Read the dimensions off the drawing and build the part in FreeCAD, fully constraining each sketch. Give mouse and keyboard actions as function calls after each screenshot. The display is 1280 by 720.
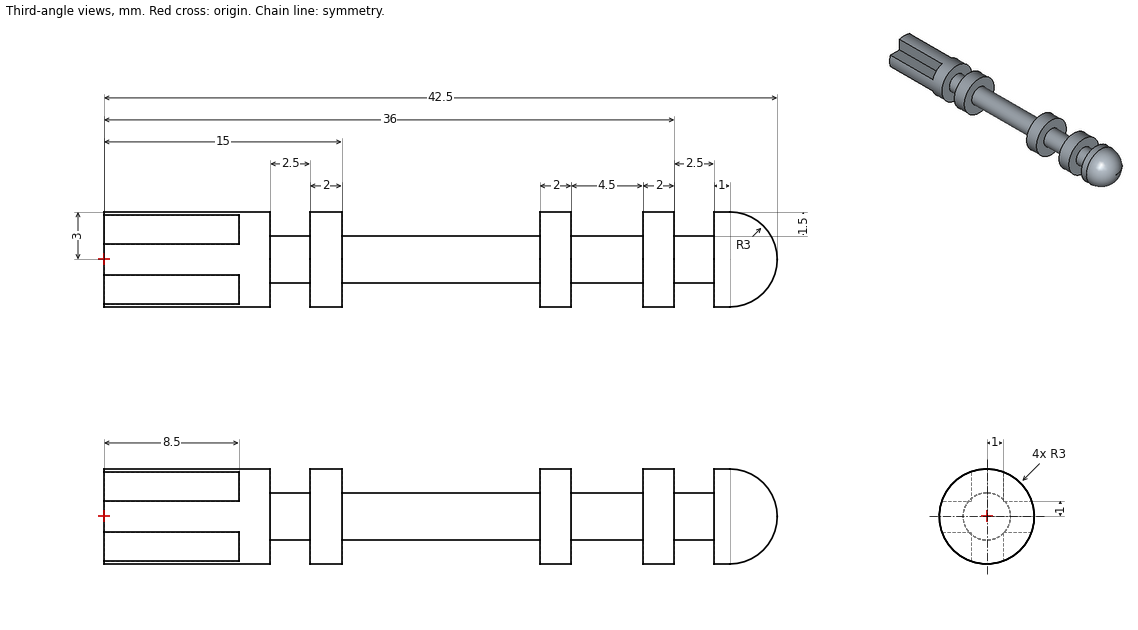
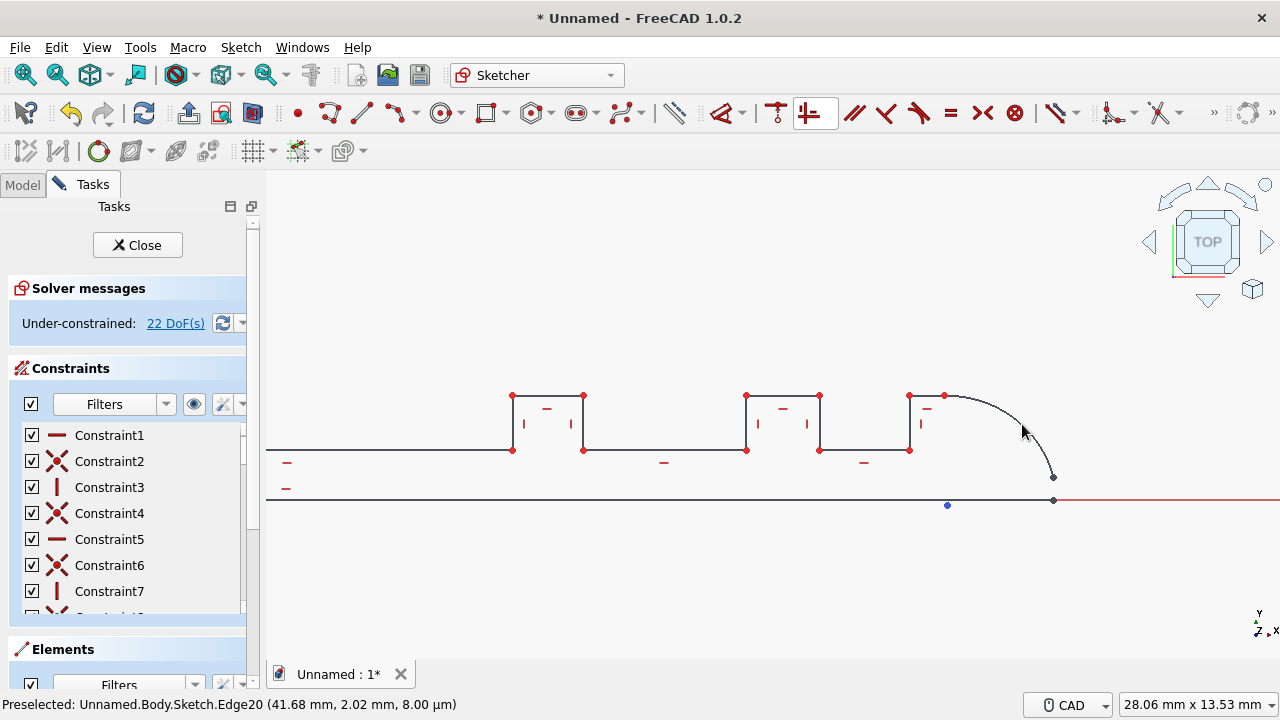
scroll(934, 396, up, 2)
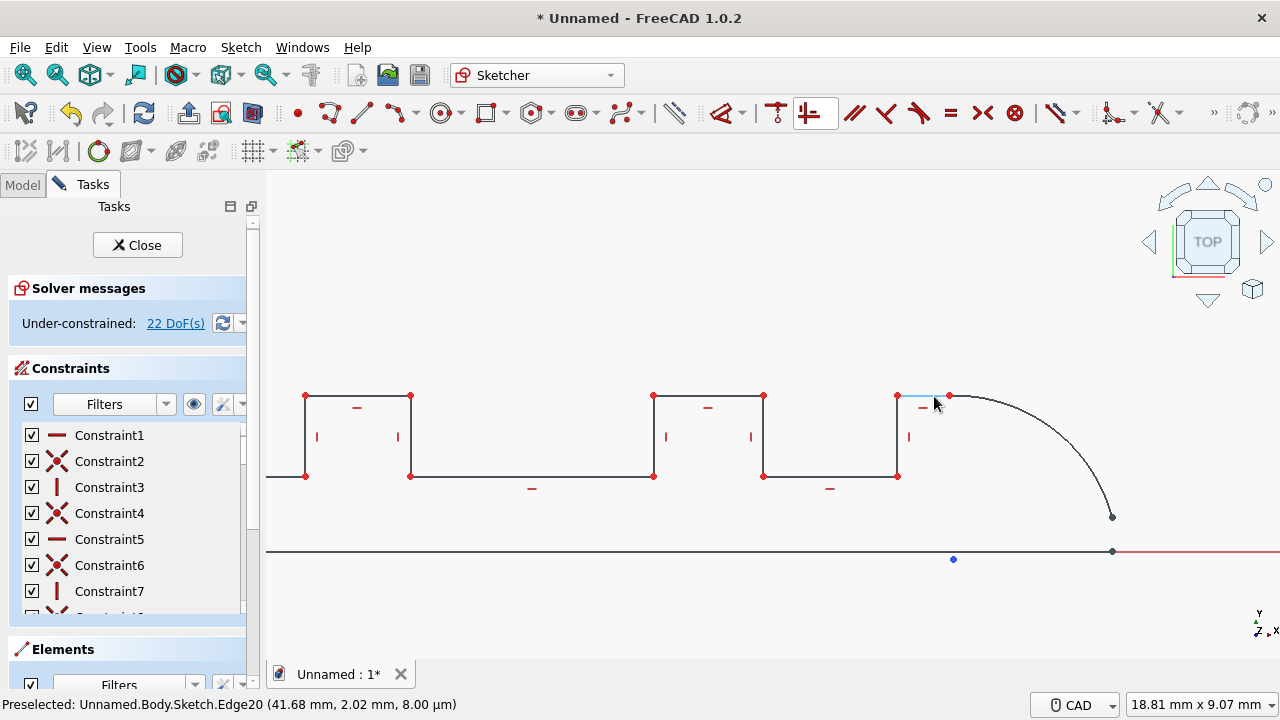
click(934, 396)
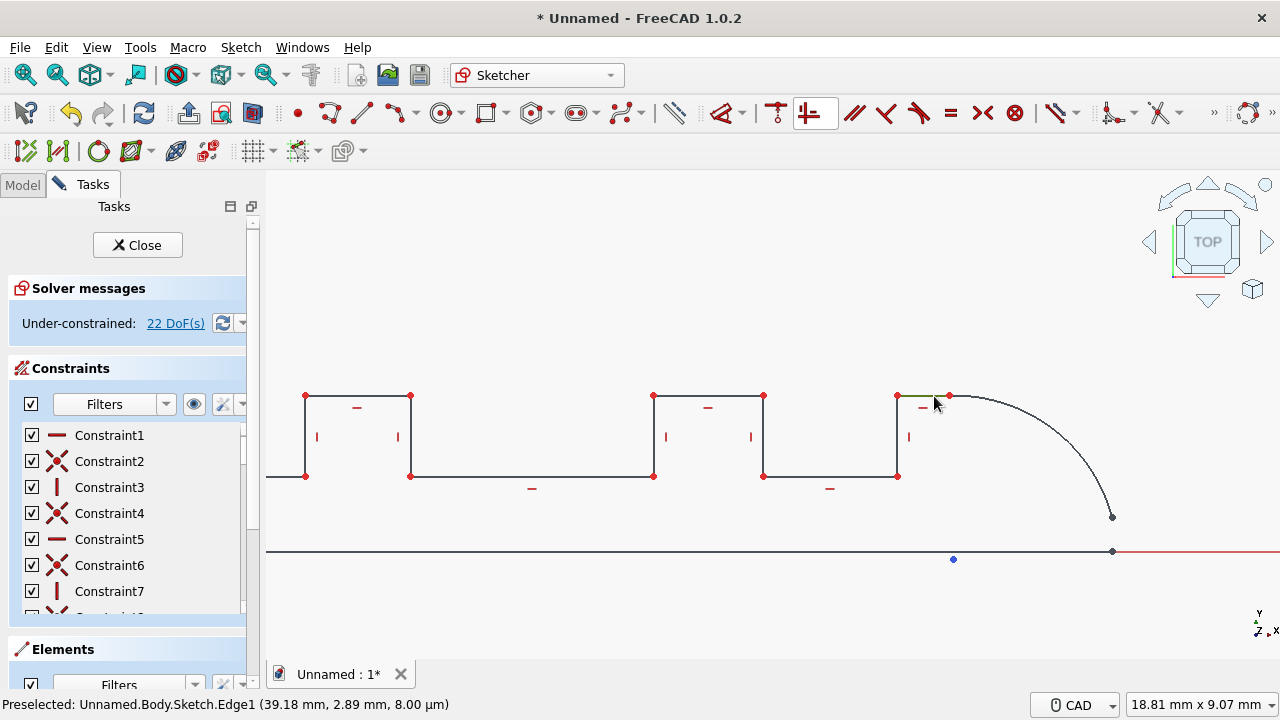
scroll(946, 396, down, 7)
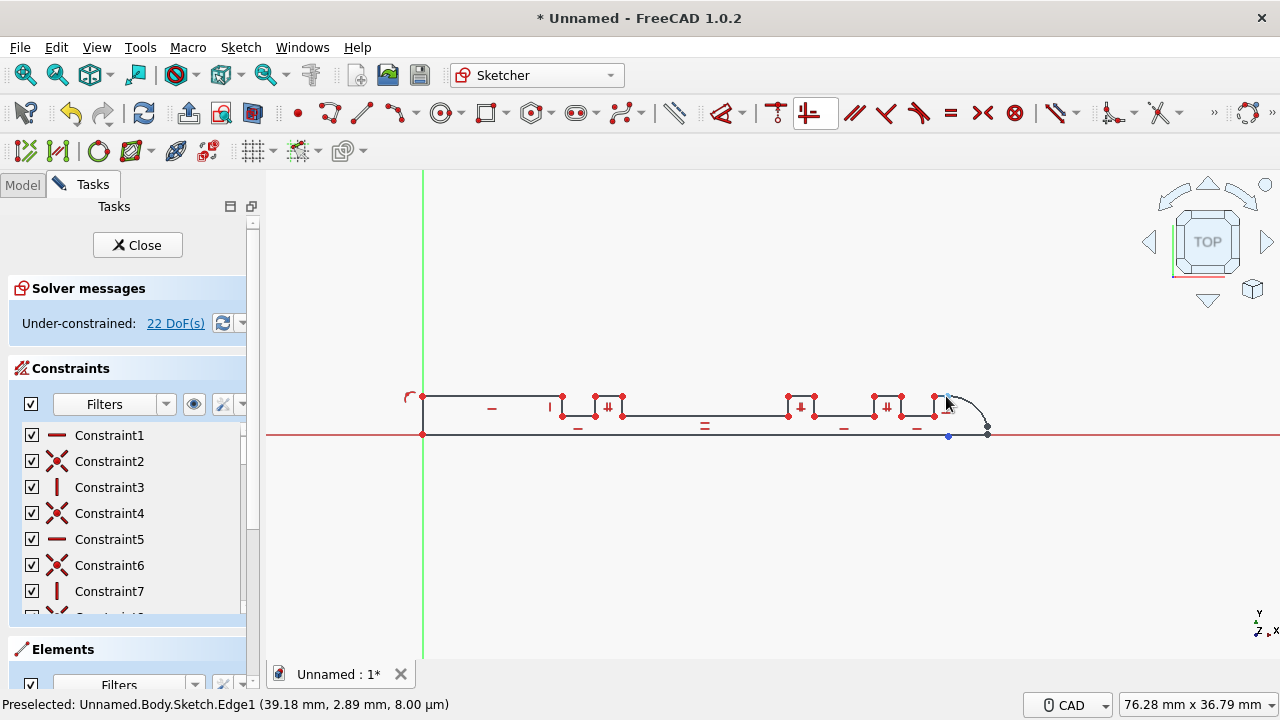
click(980, 412)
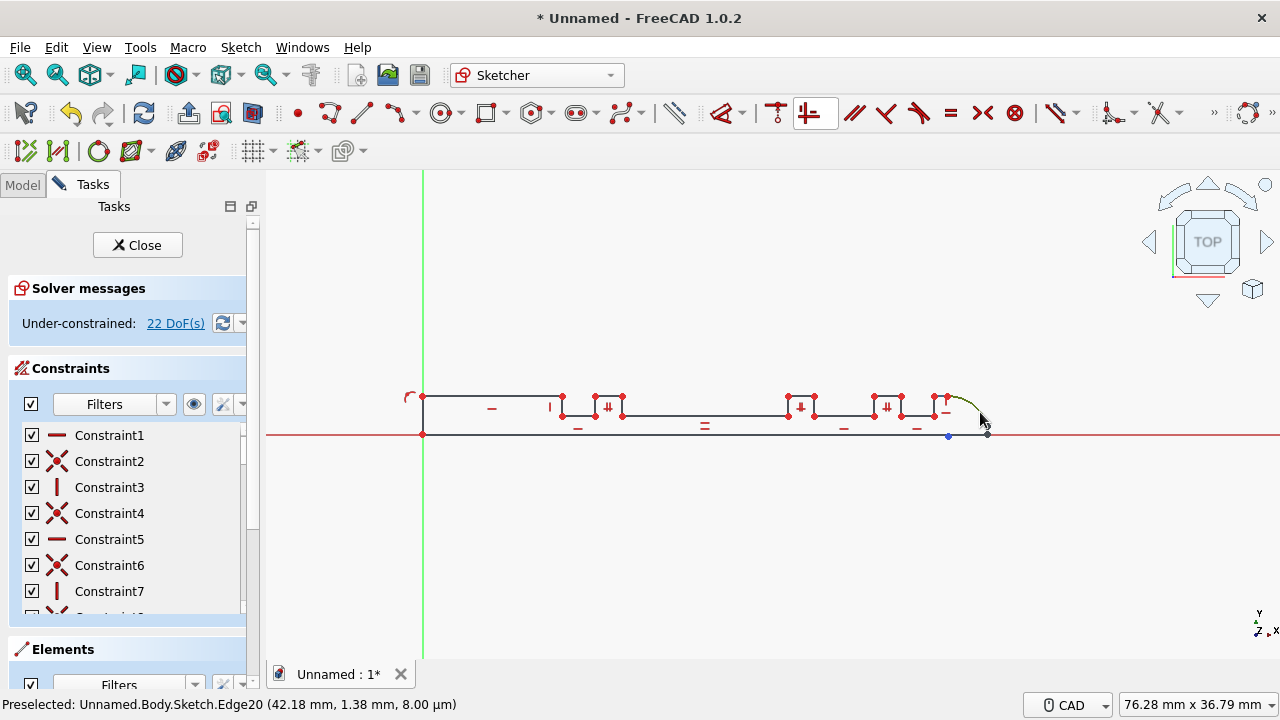
click(920, 114)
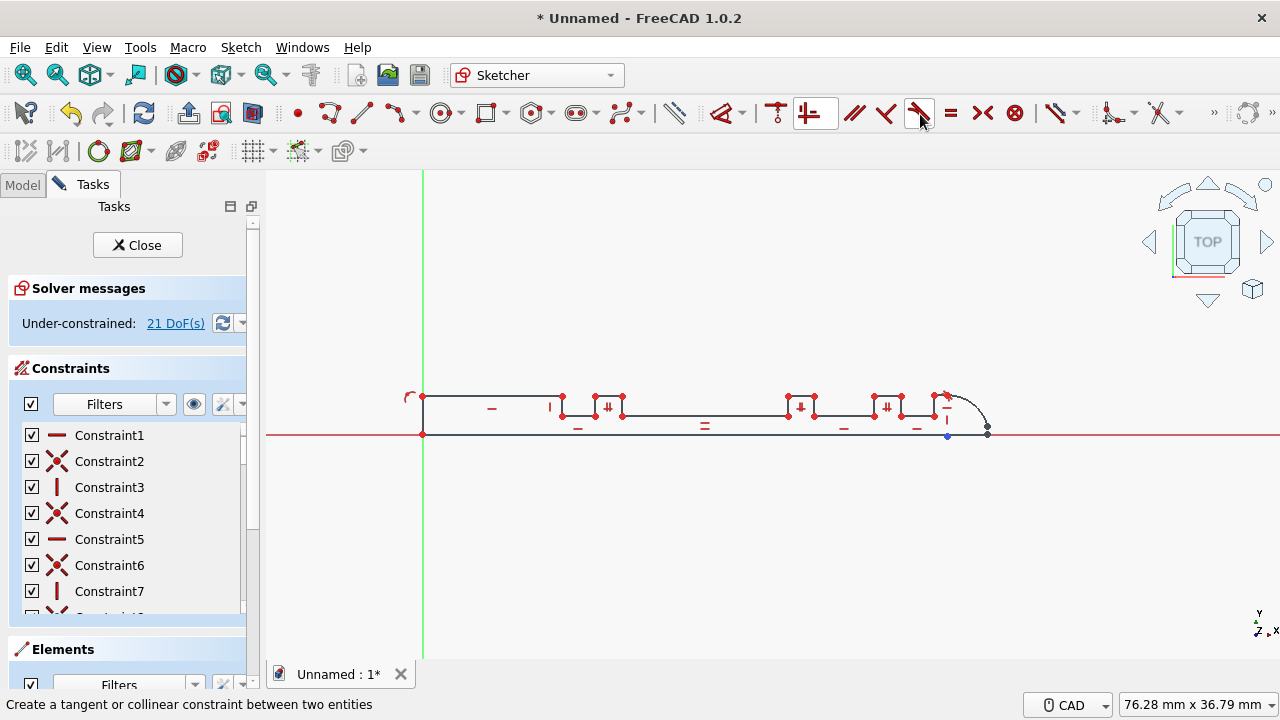
click(947, 437)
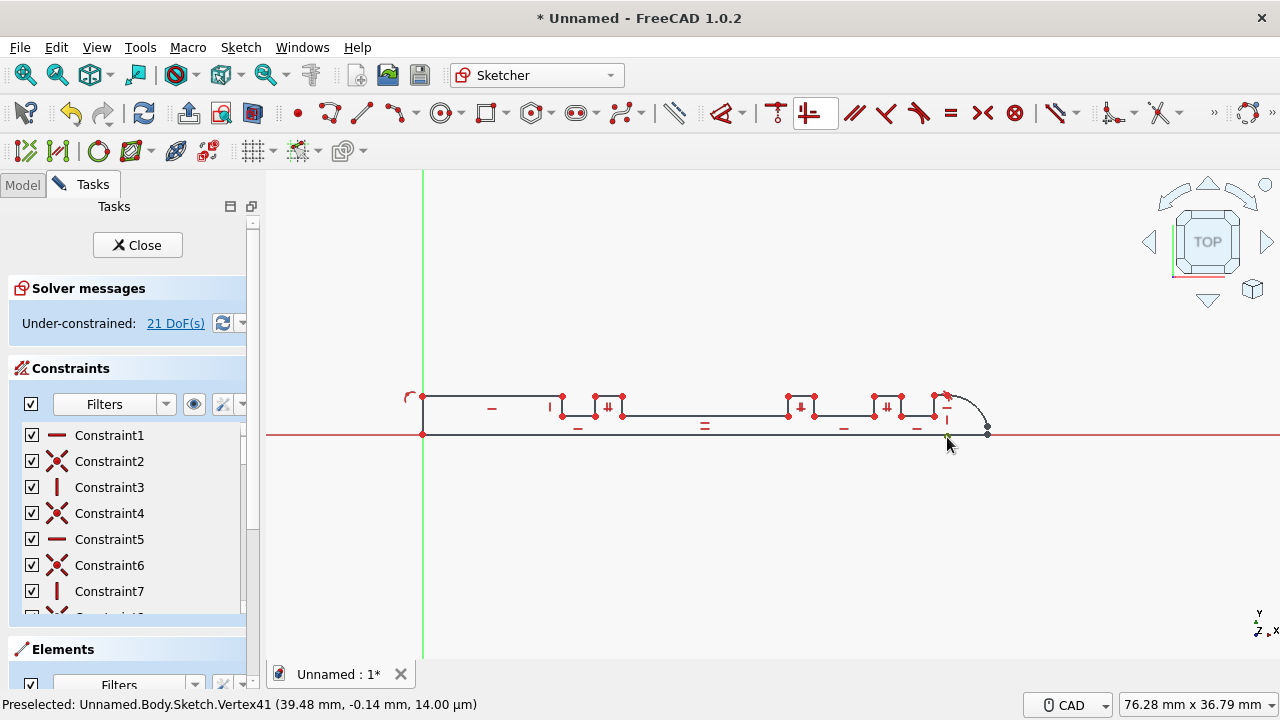
click(353, 435)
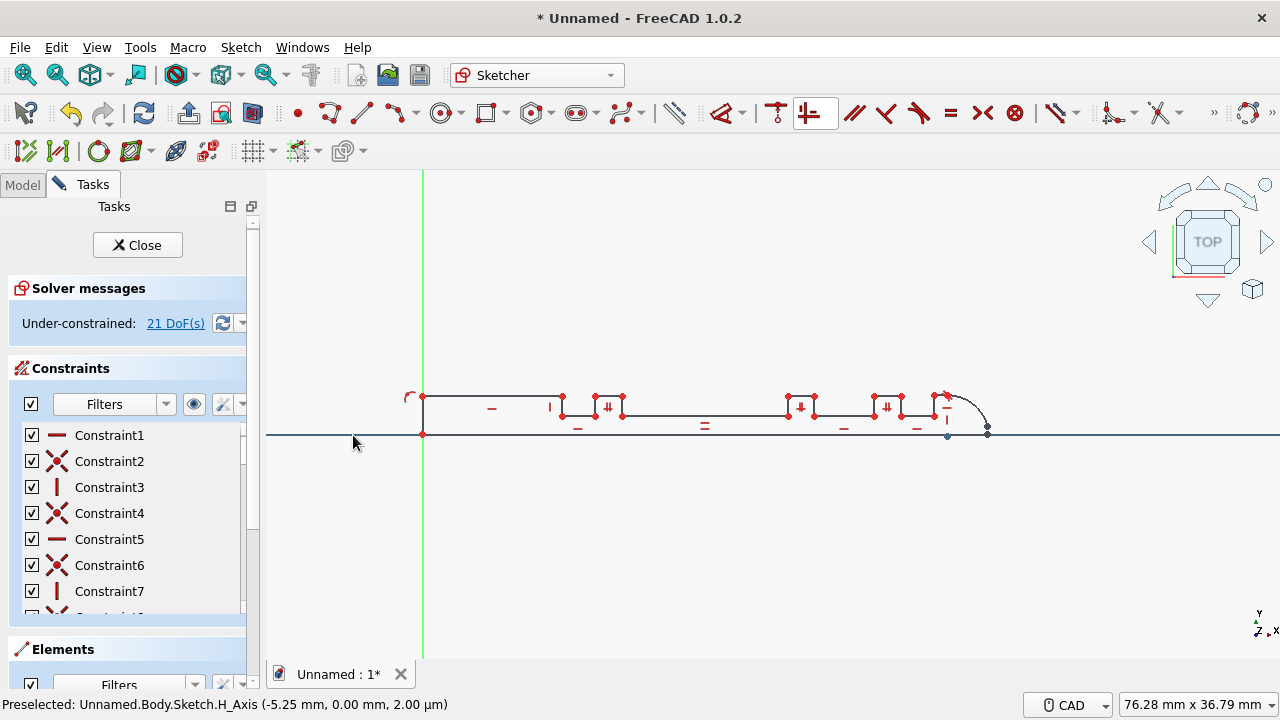
click(776, 114)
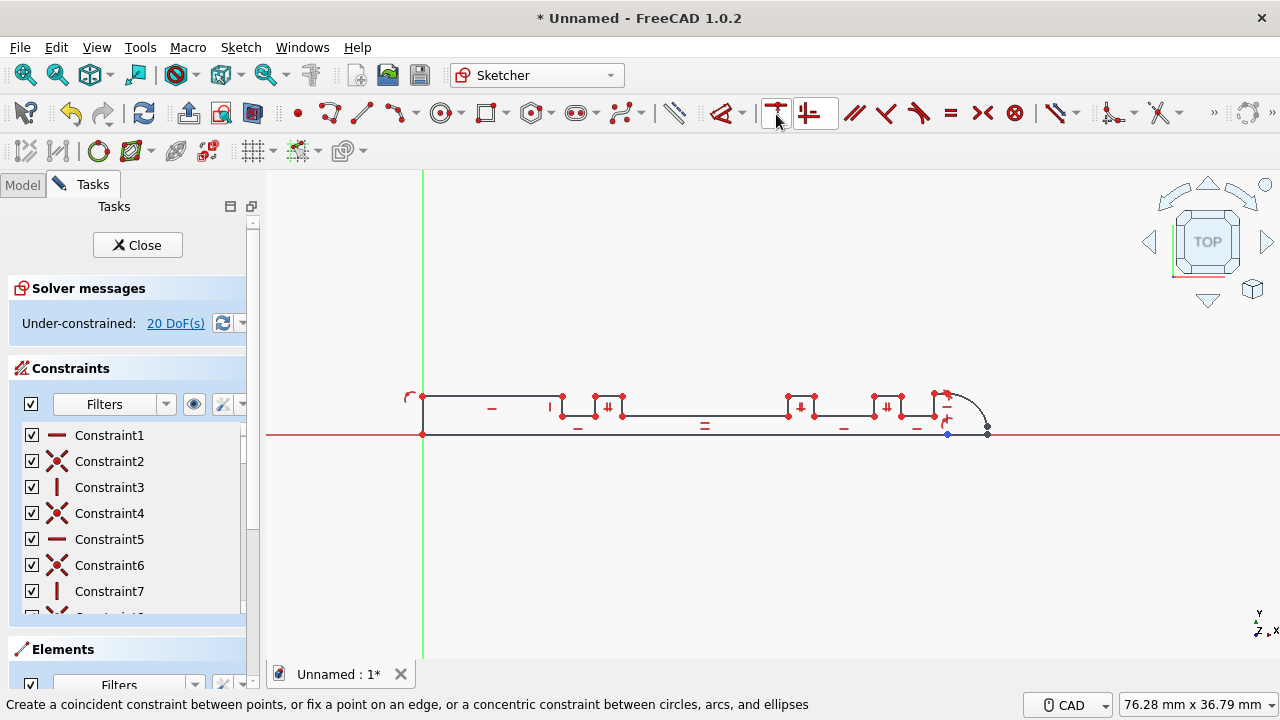
click(722, 114)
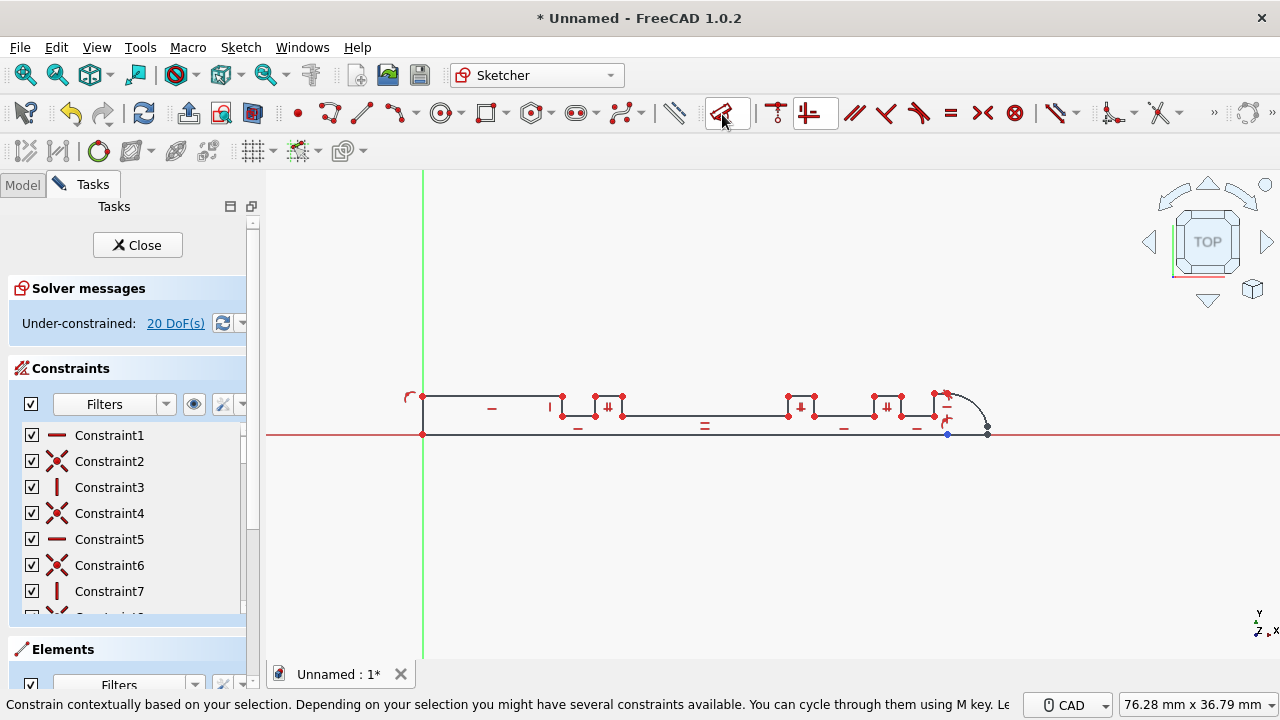
click(981, 411)
click(1007, 393)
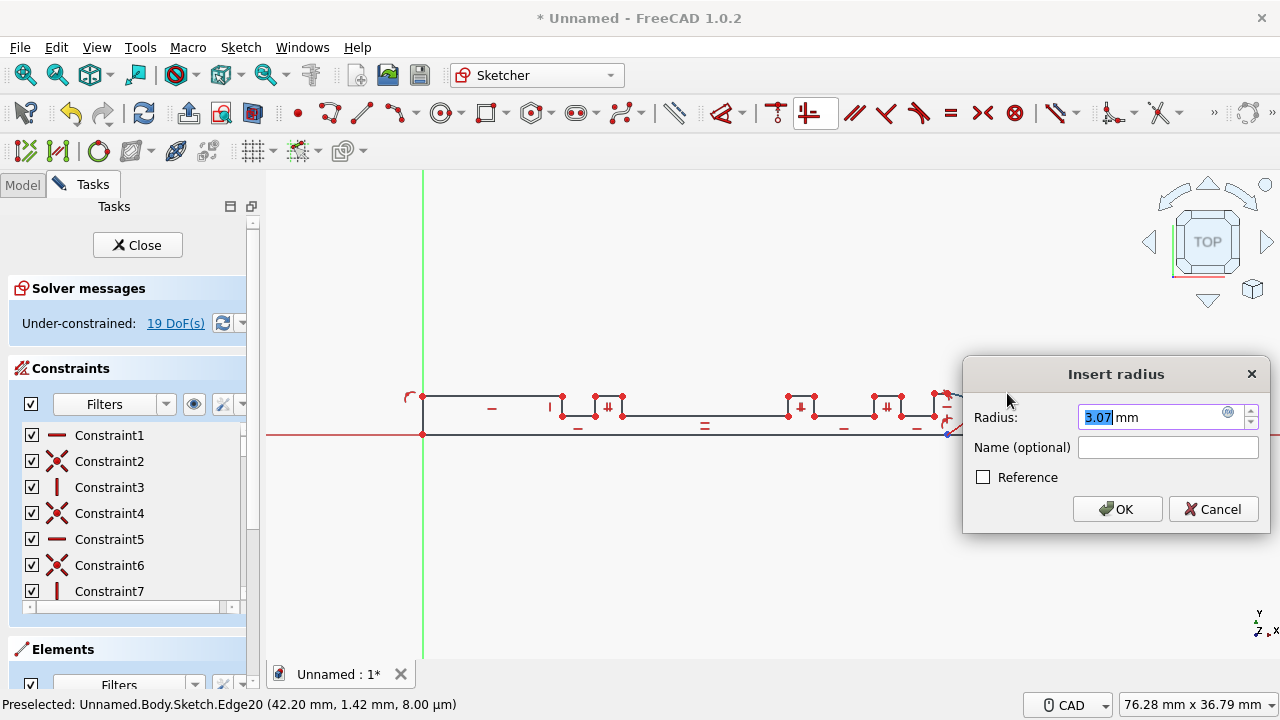
text(3)
key(Return)
key(Escape)